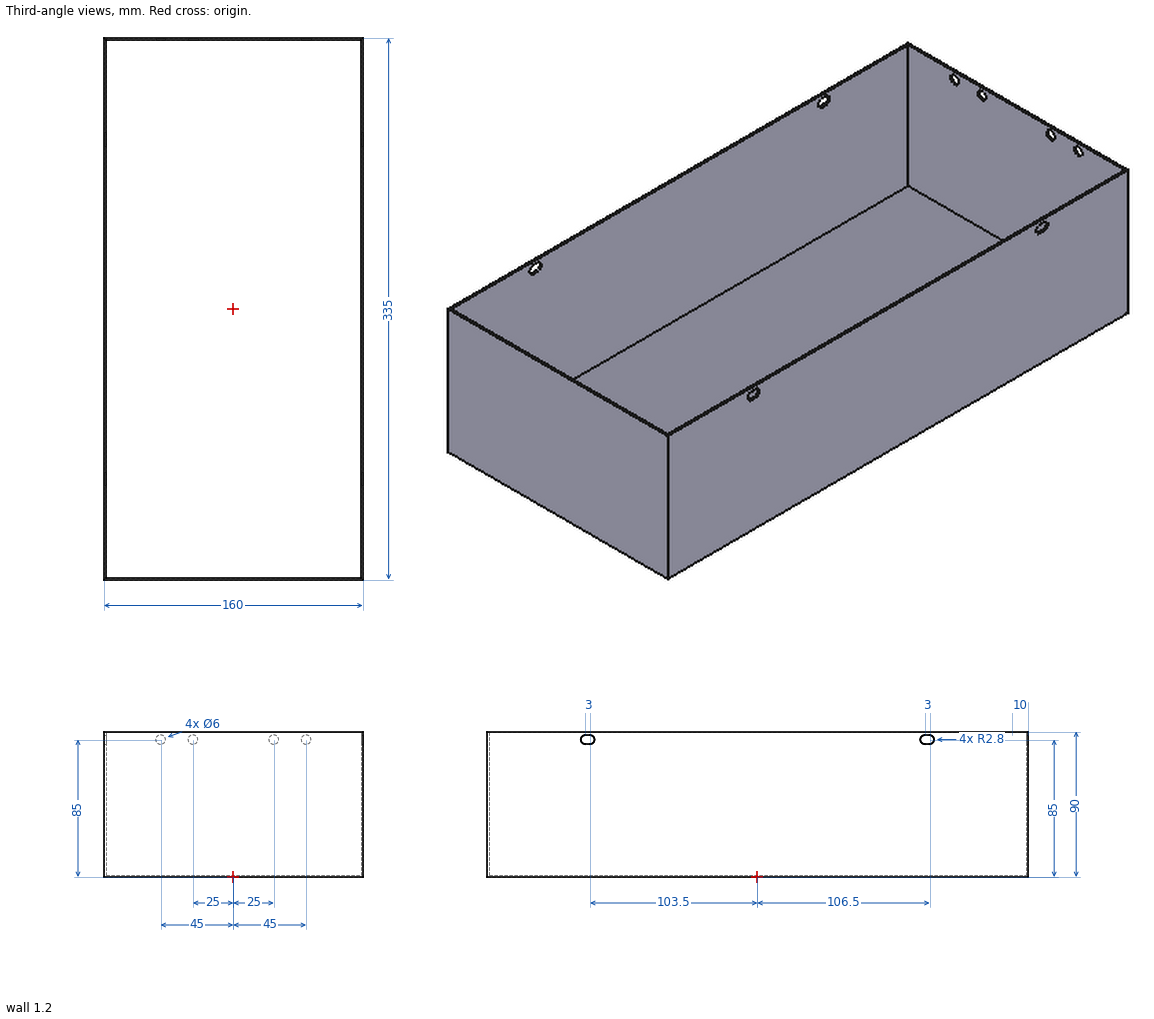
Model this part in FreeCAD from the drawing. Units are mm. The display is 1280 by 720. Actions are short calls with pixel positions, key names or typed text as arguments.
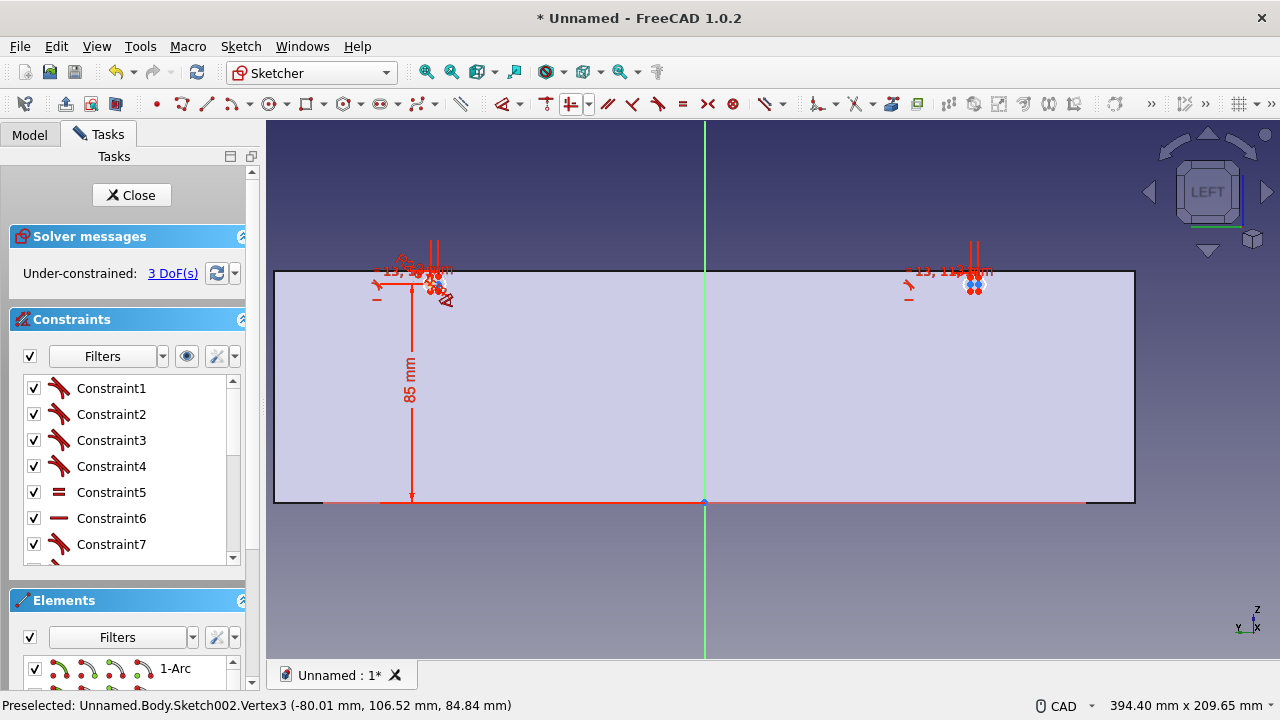
scroll(971, 284, up, 3)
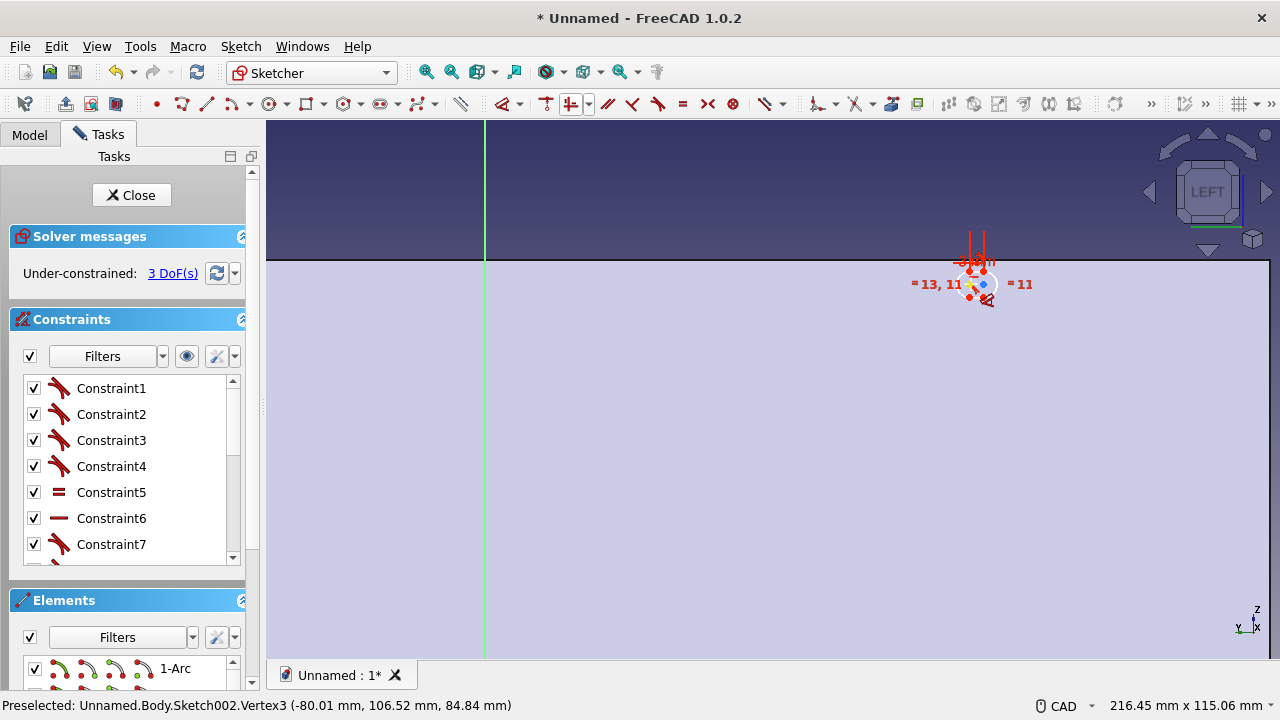
click(970, 285)
click(1004, 458)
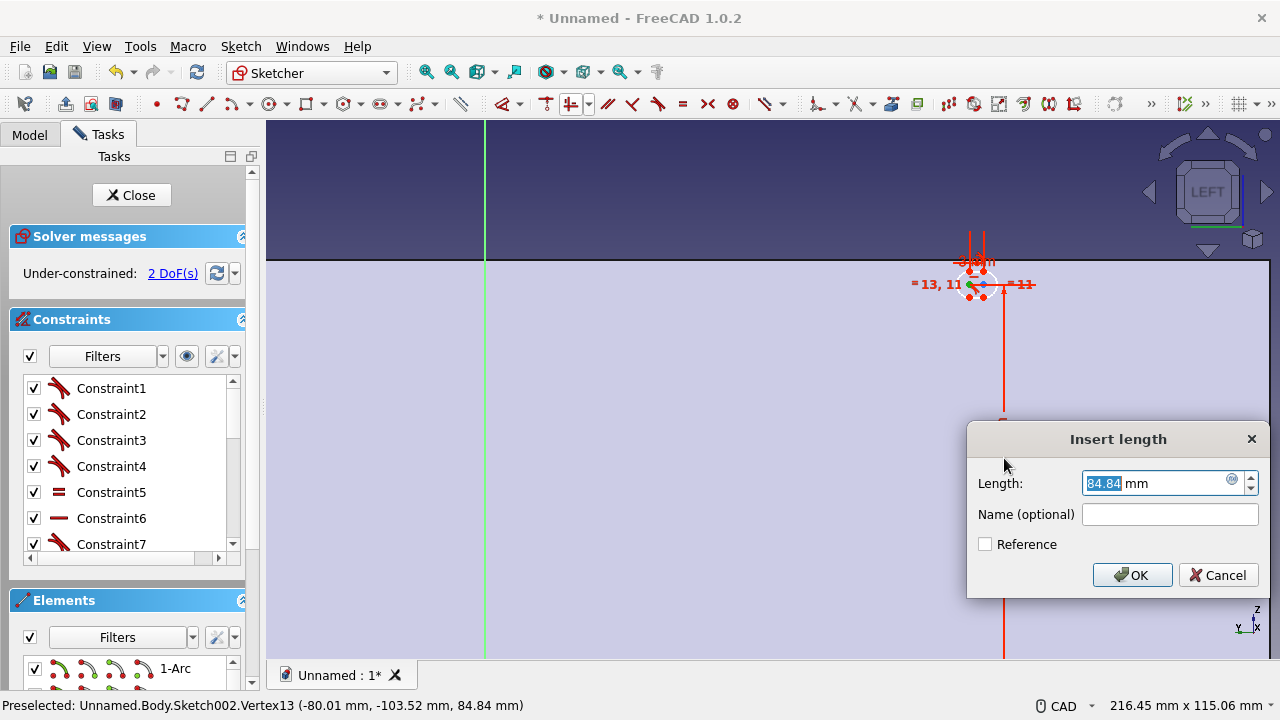
text(85)
key(Return)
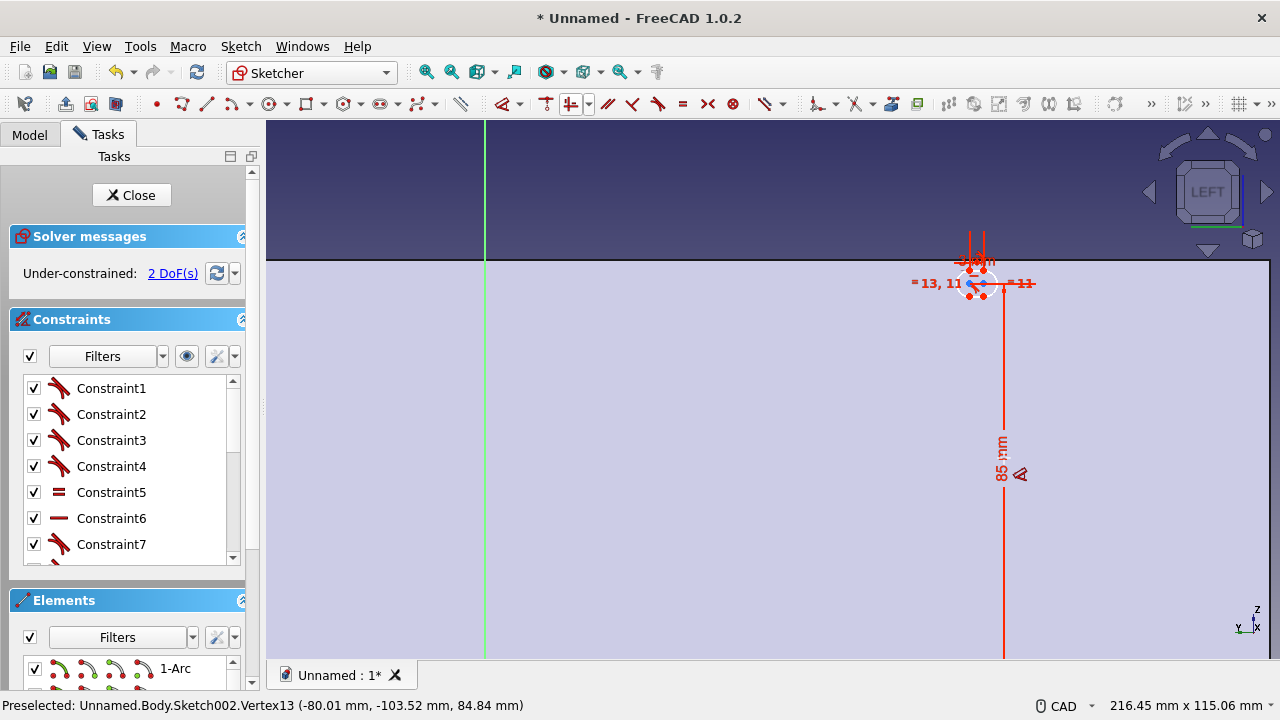
scroll(972, 284, down, 3)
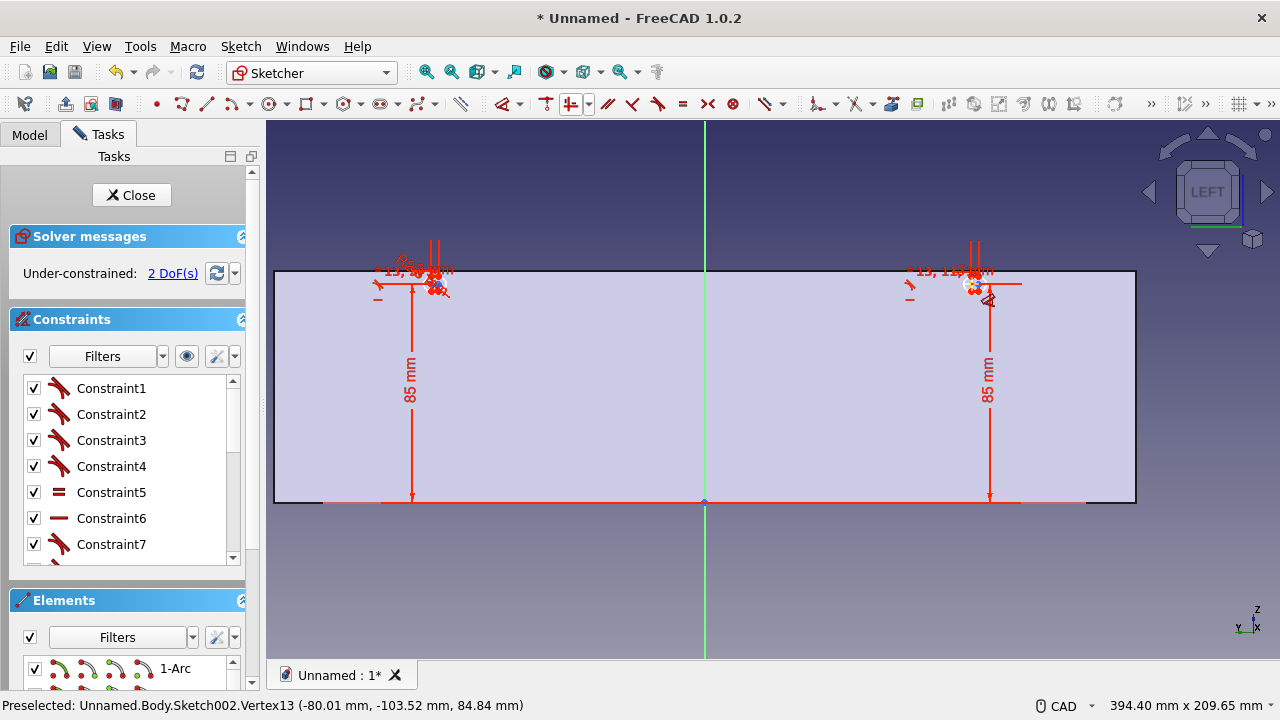
scroll(431, 277, up, 3)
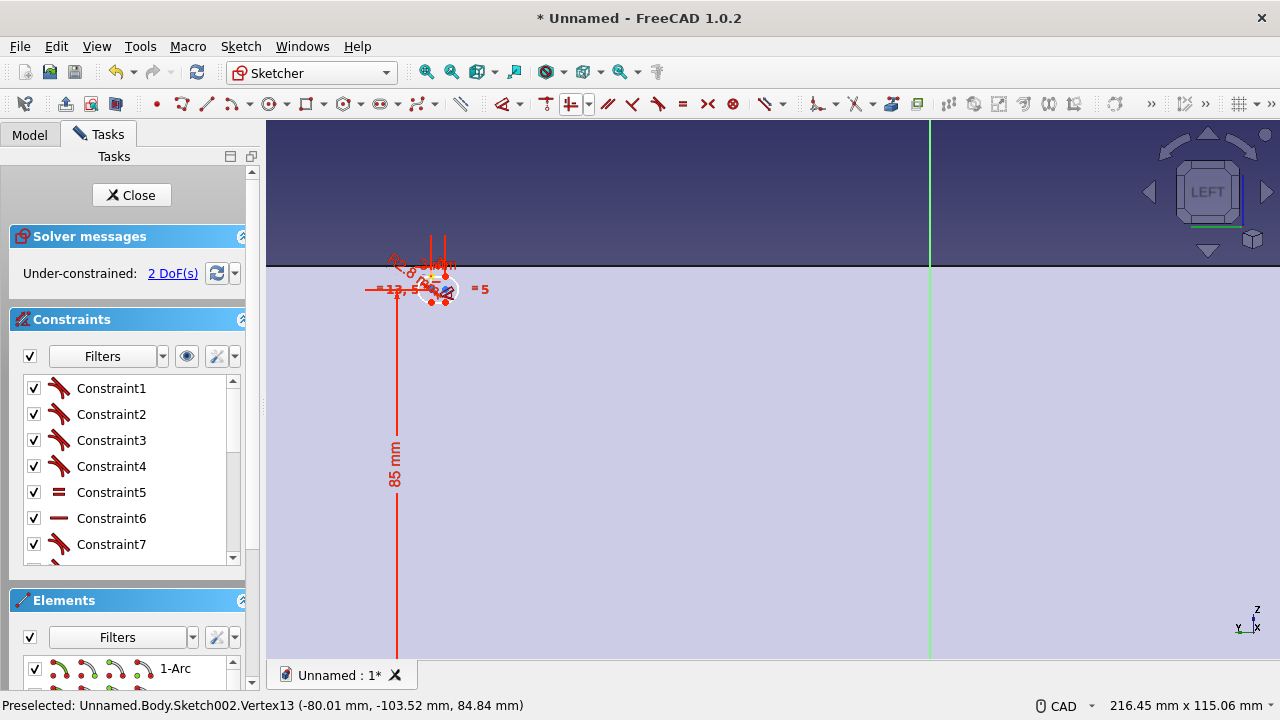
click(431, 277)
click(681, 243)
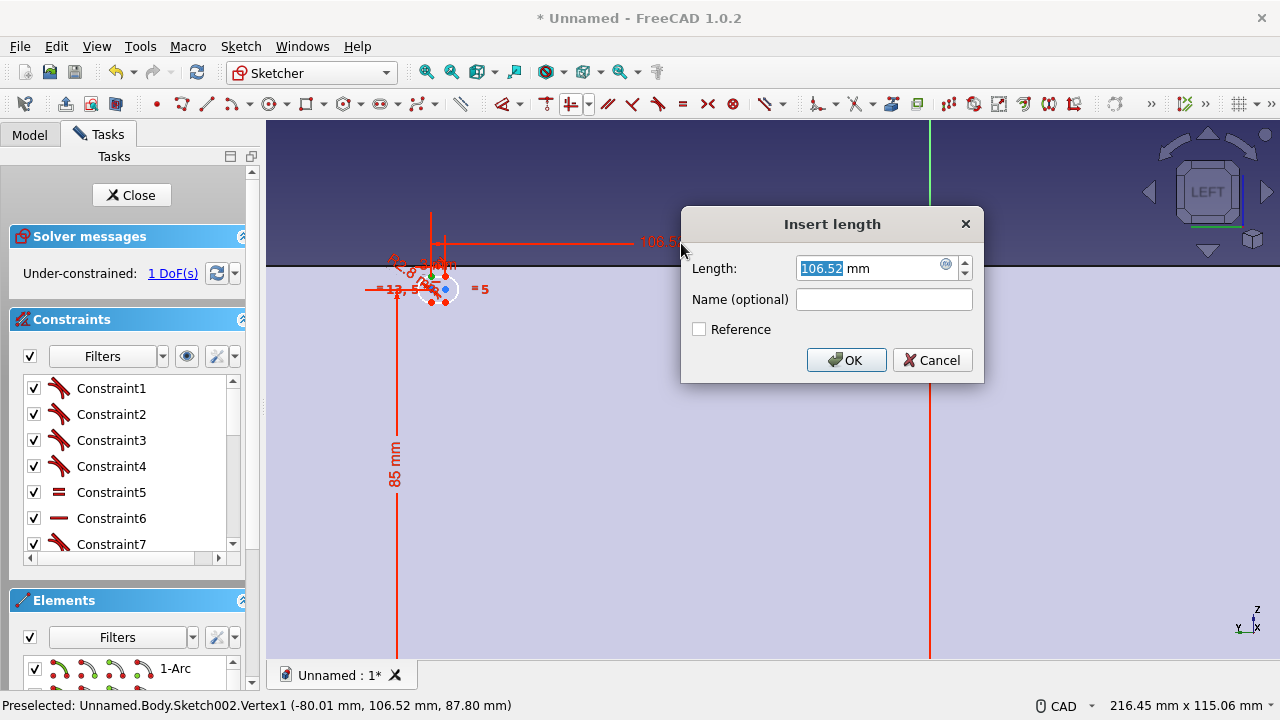
text(106.5)
key(Return)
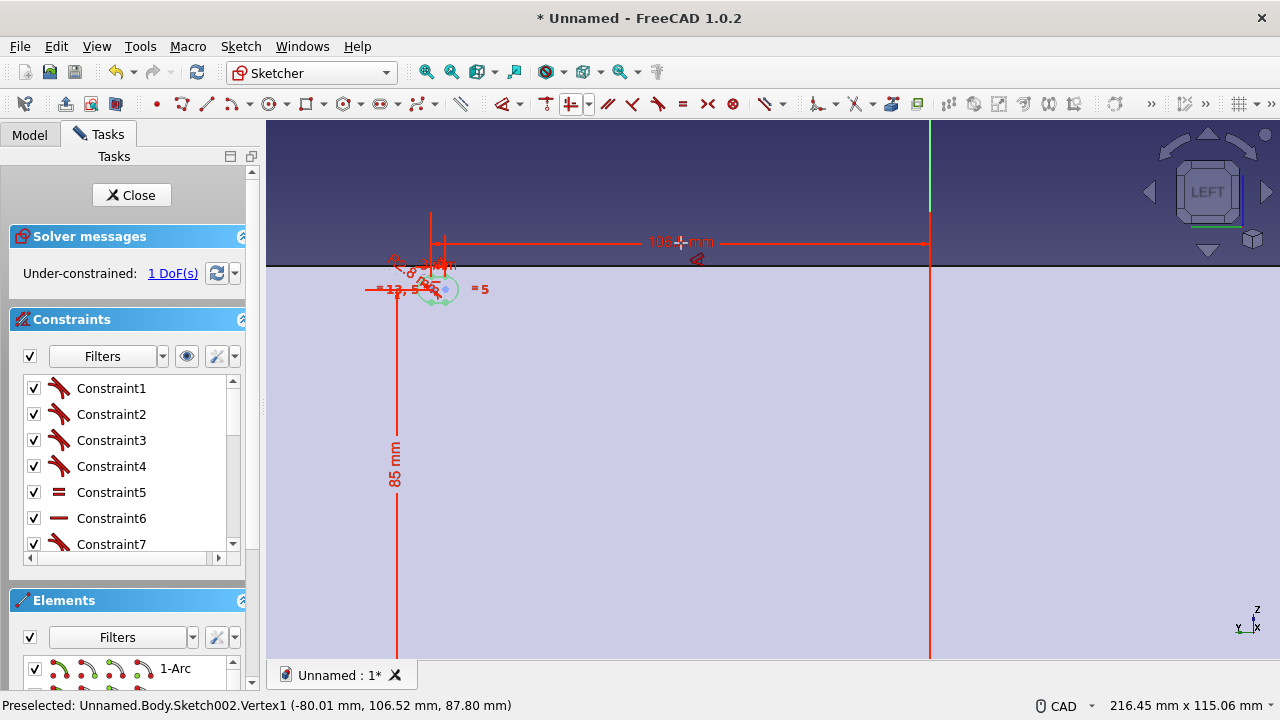
scroll(430, 277, down, 3)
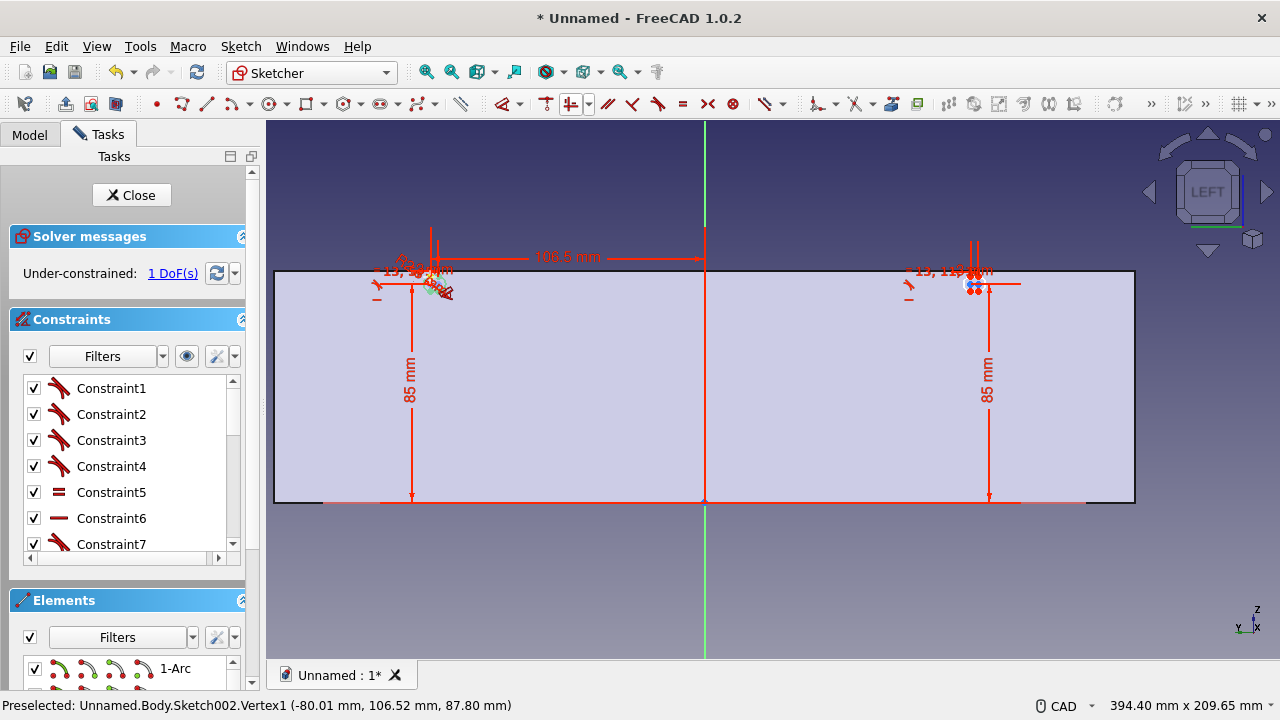
scroll(971, 277, up, 3)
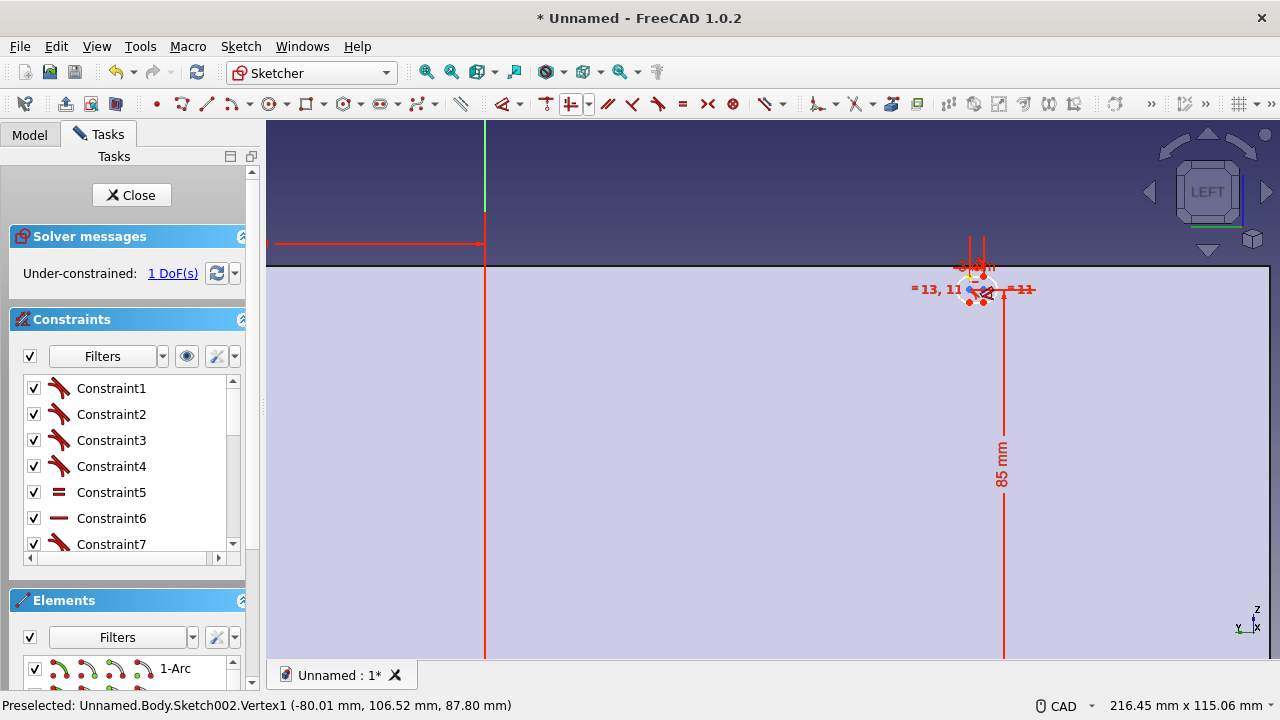
click(970, 277)
click(727, 243)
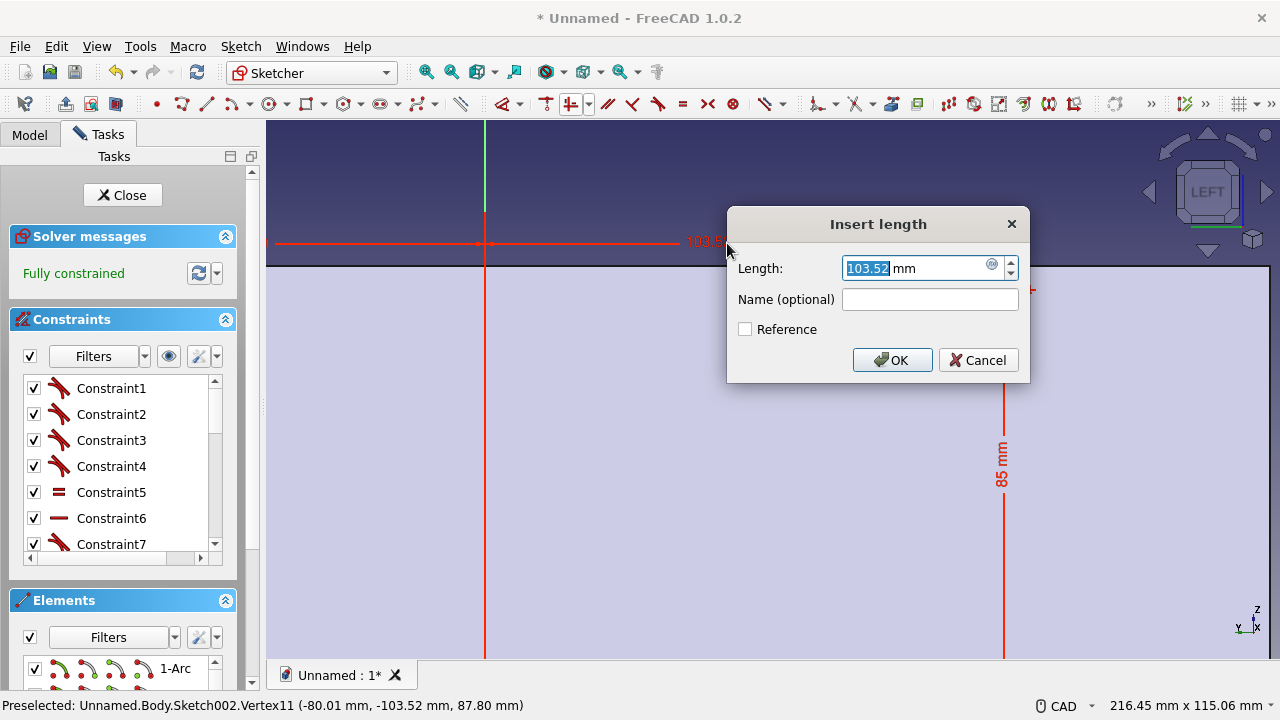
text(103.5)
key(Return)
key(Escape)